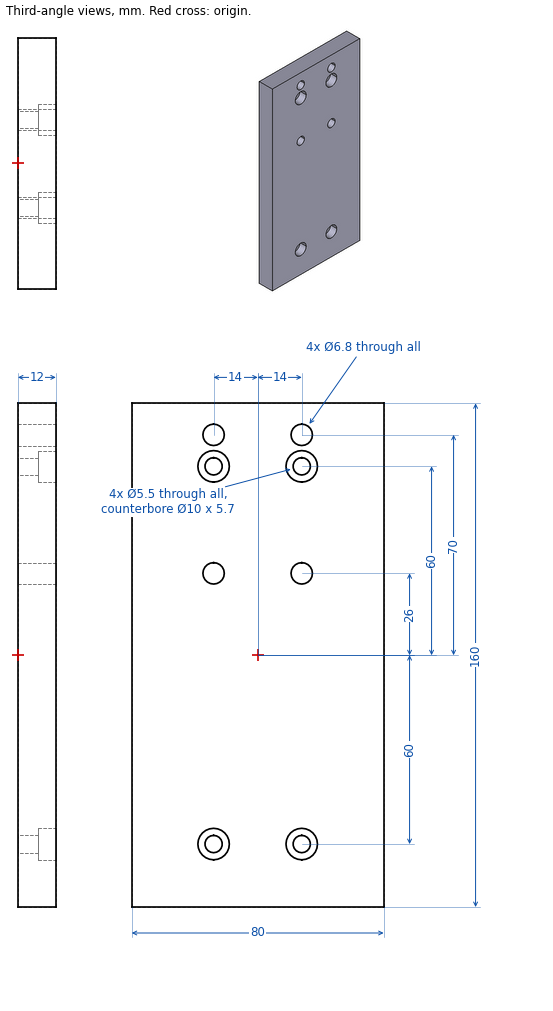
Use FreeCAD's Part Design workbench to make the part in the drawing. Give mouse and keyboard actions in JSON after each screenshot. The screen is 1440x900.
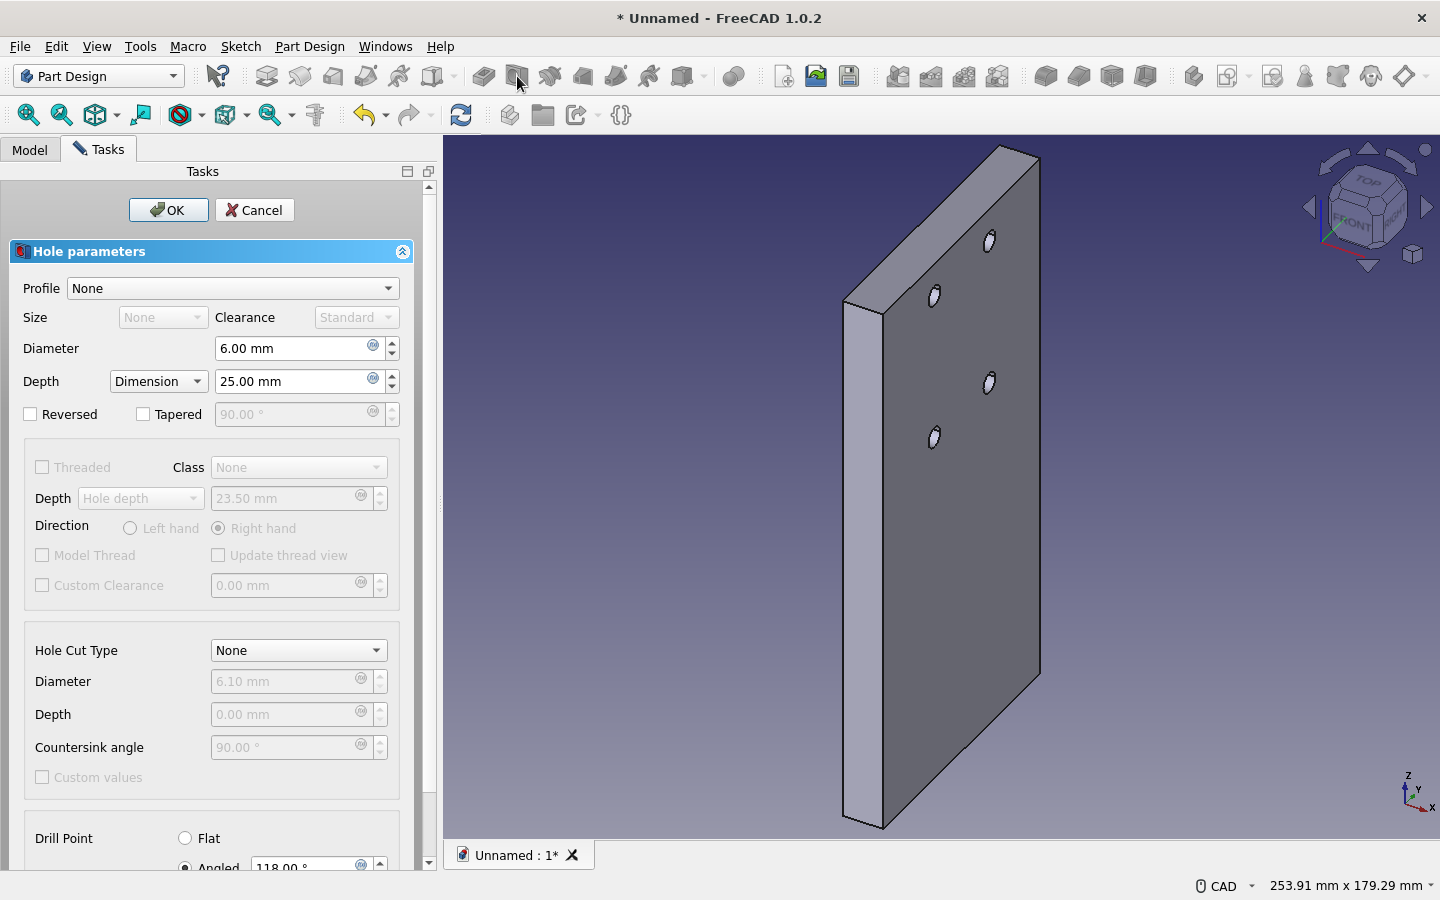
{"action": "triple_click", "coordinate": [300, 348]}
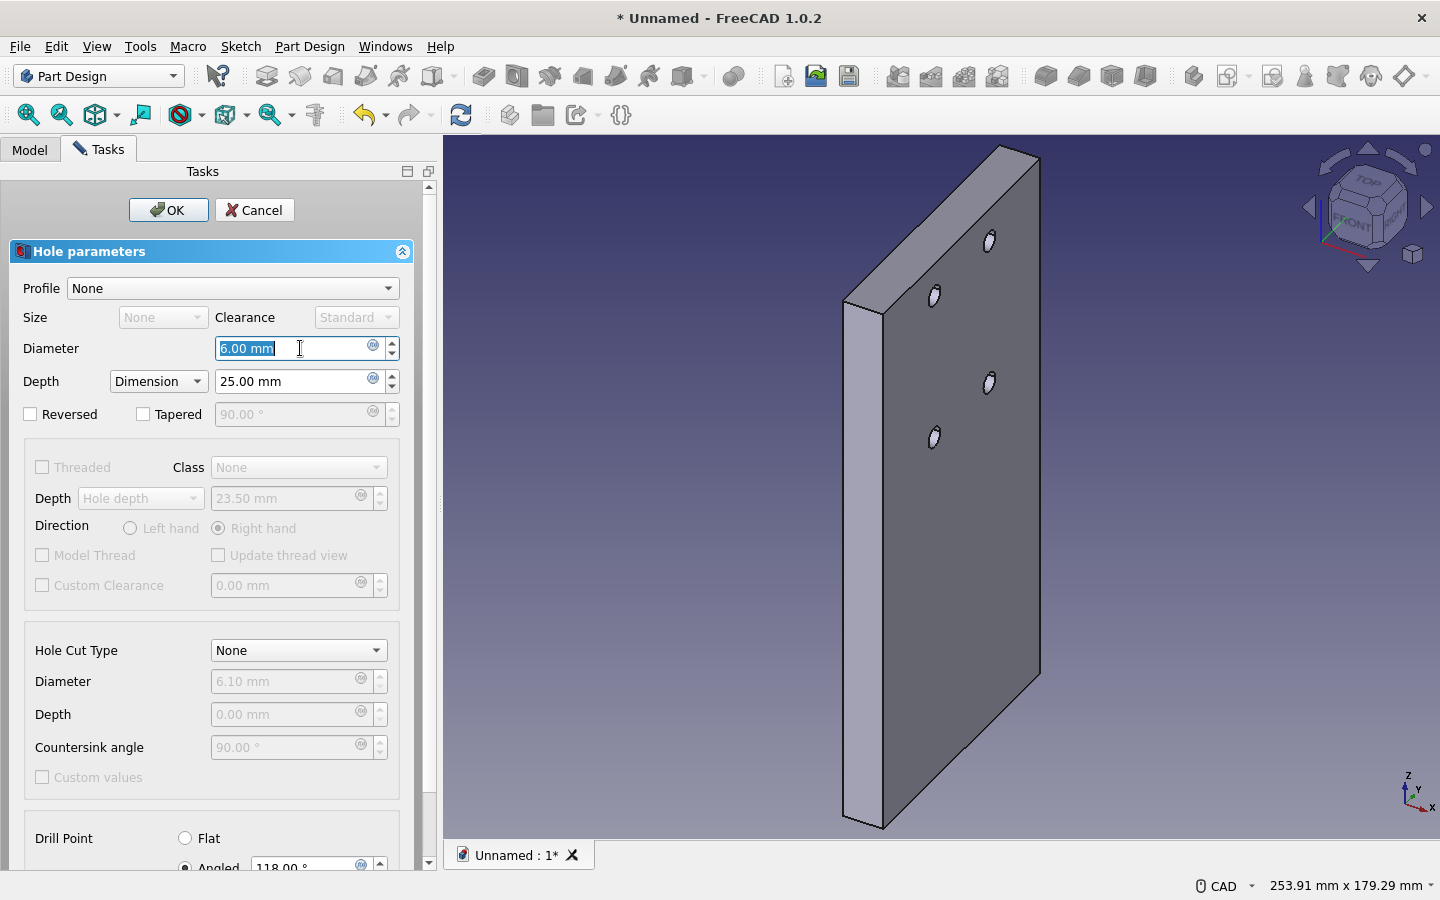
{"action": "type", "text": "6.8"}
{"action": "key", "text": "Tab"}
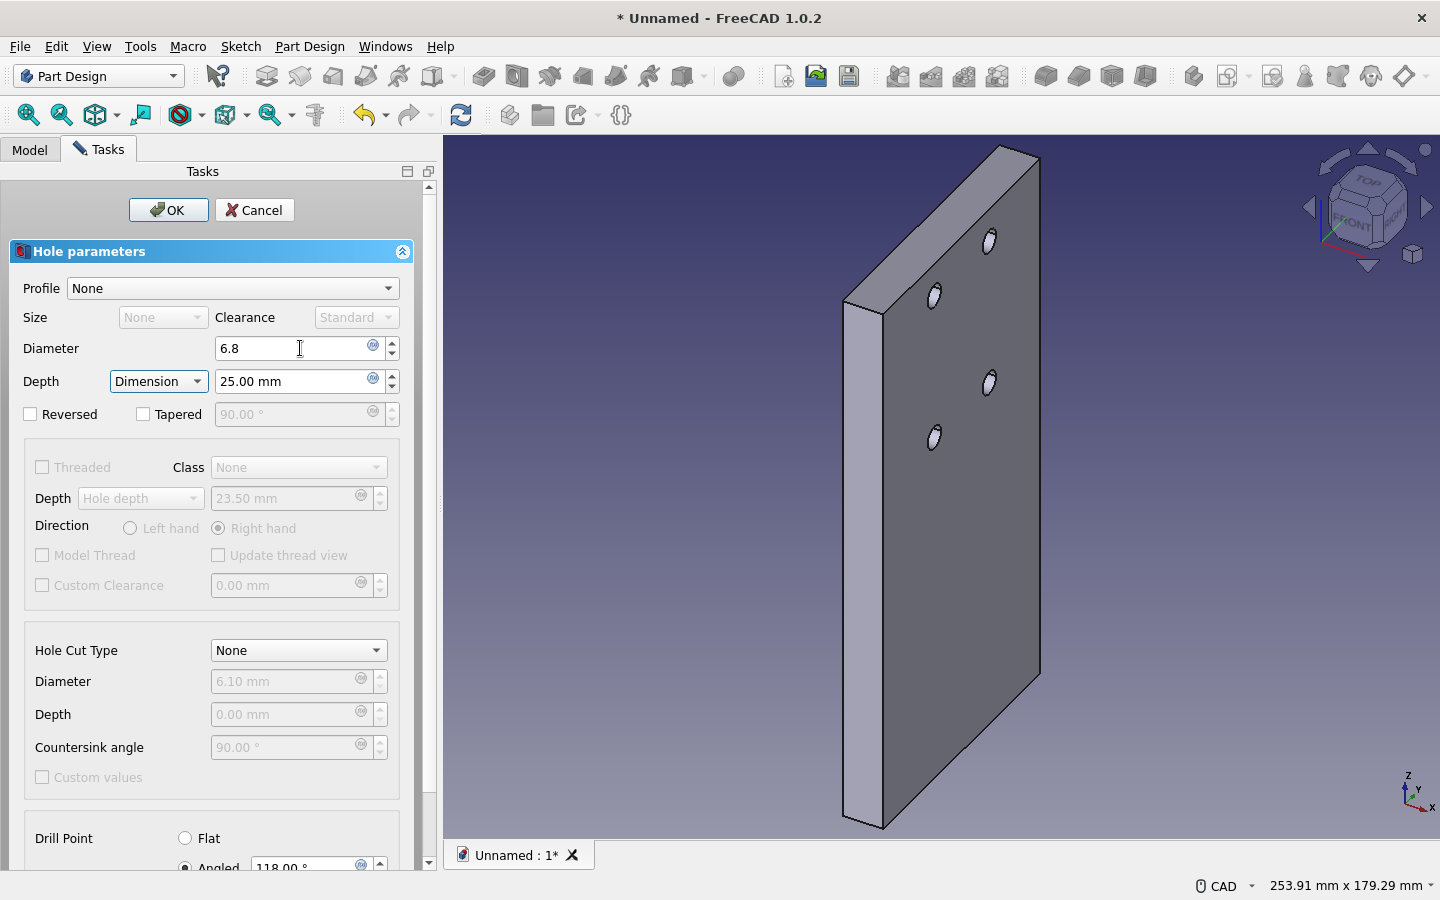
{"action": "left_click", "coordinate": [160, 382]}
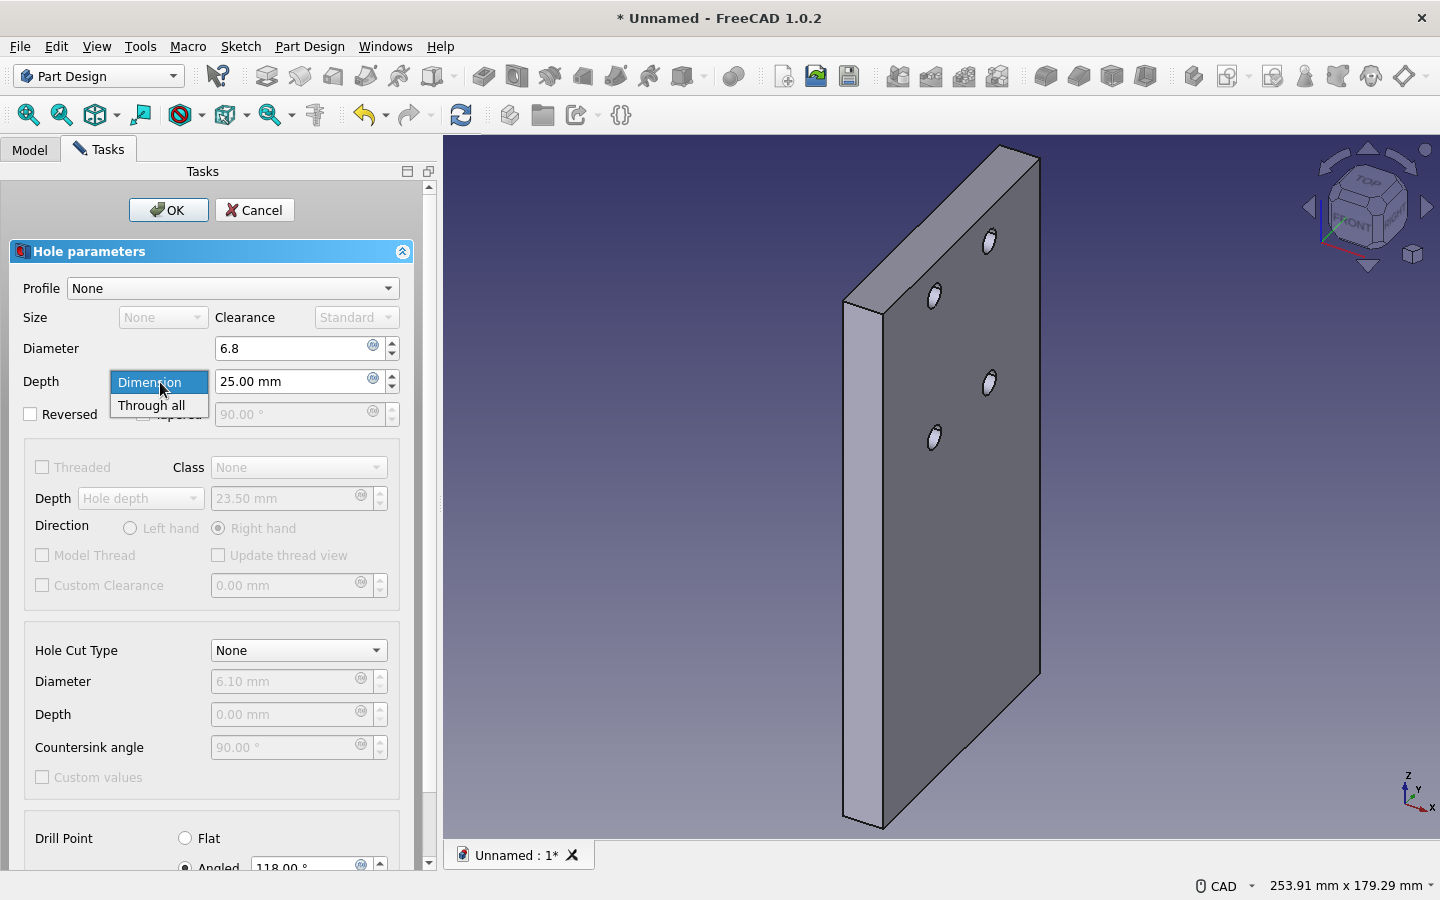
{"action": "left_click", "coordinate": [158, 406]}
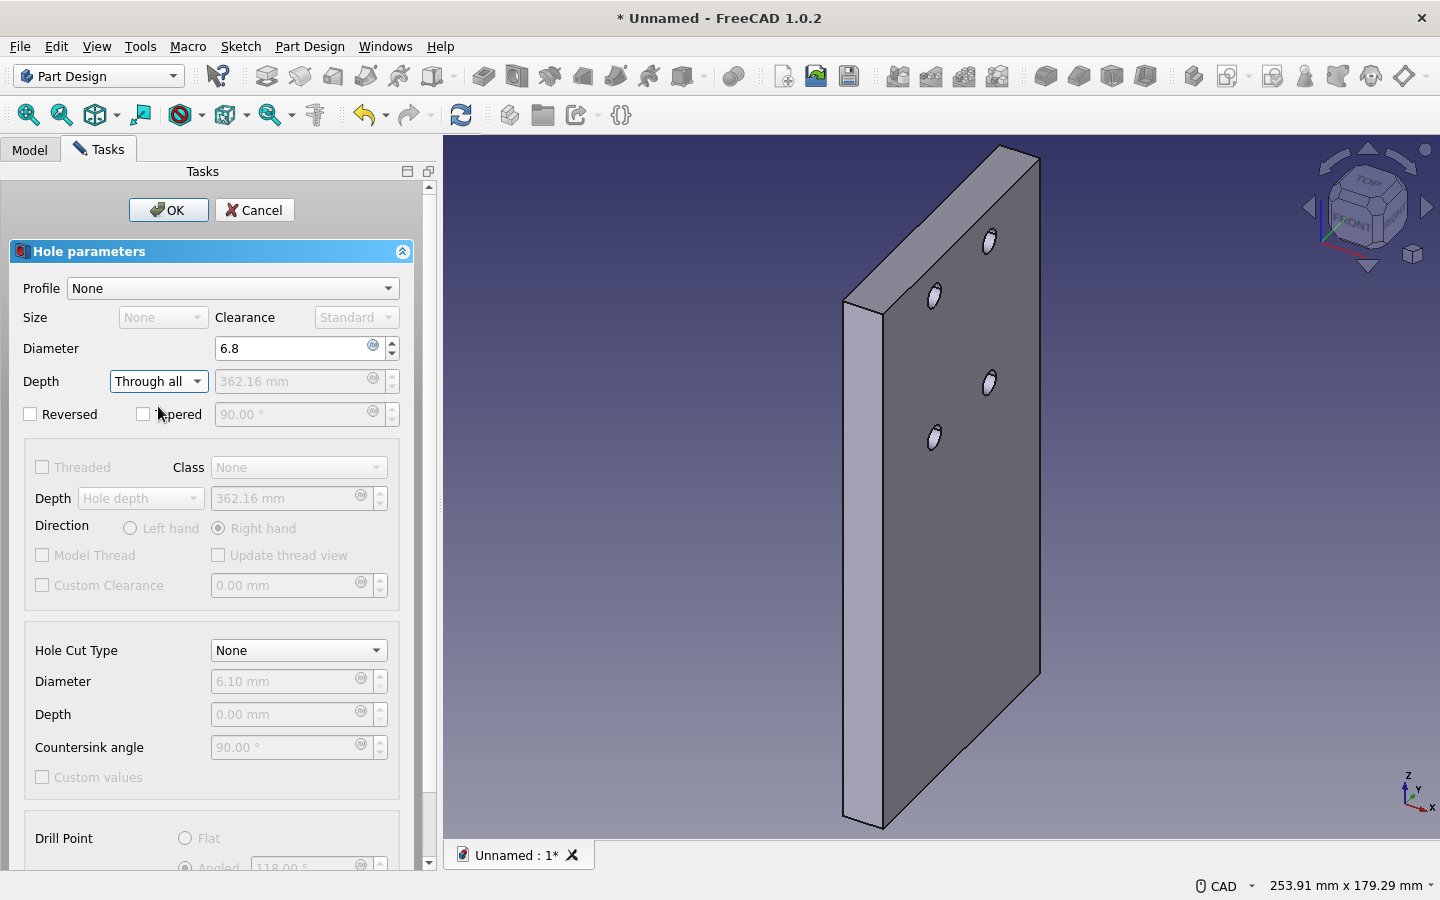
{"action": "left_click", "coordinate": [169, 210]}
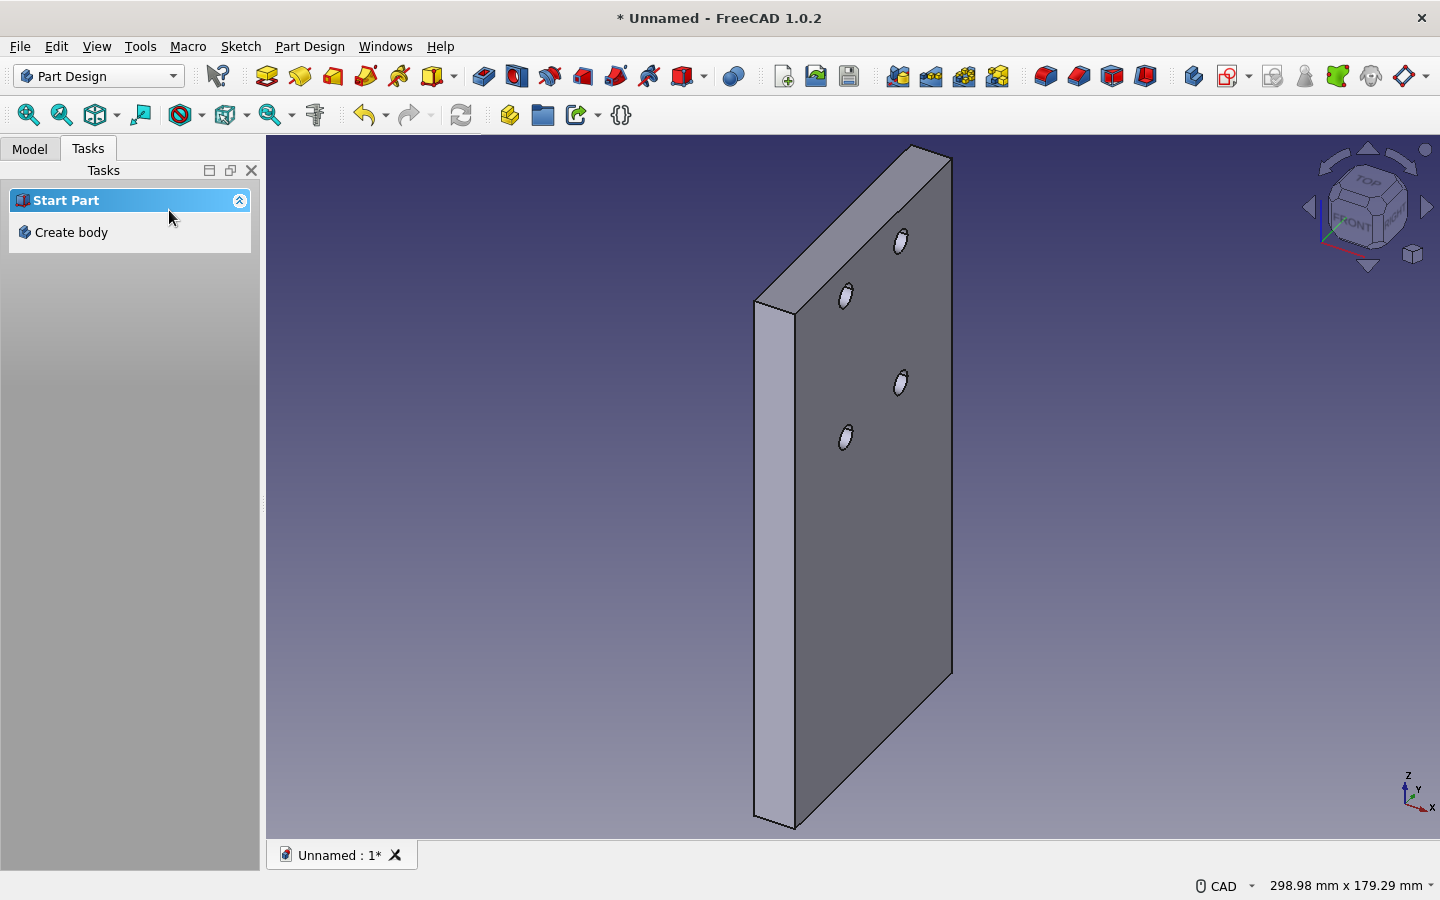
{"action": "left_click", "coordinate": [873, 566]}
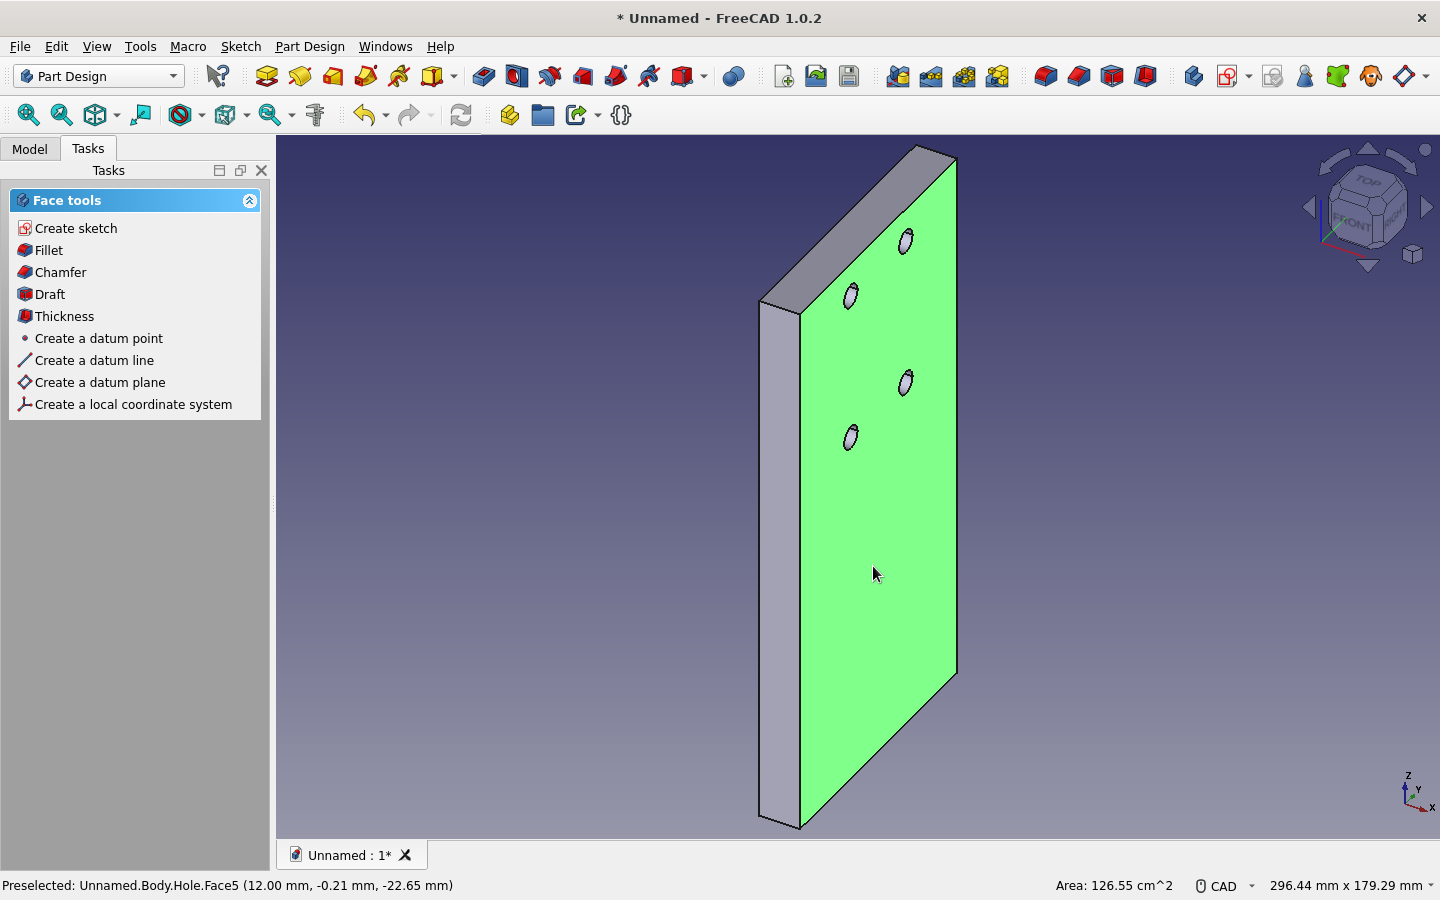
{"action": "left_click", "coordinate": [1226, 76]}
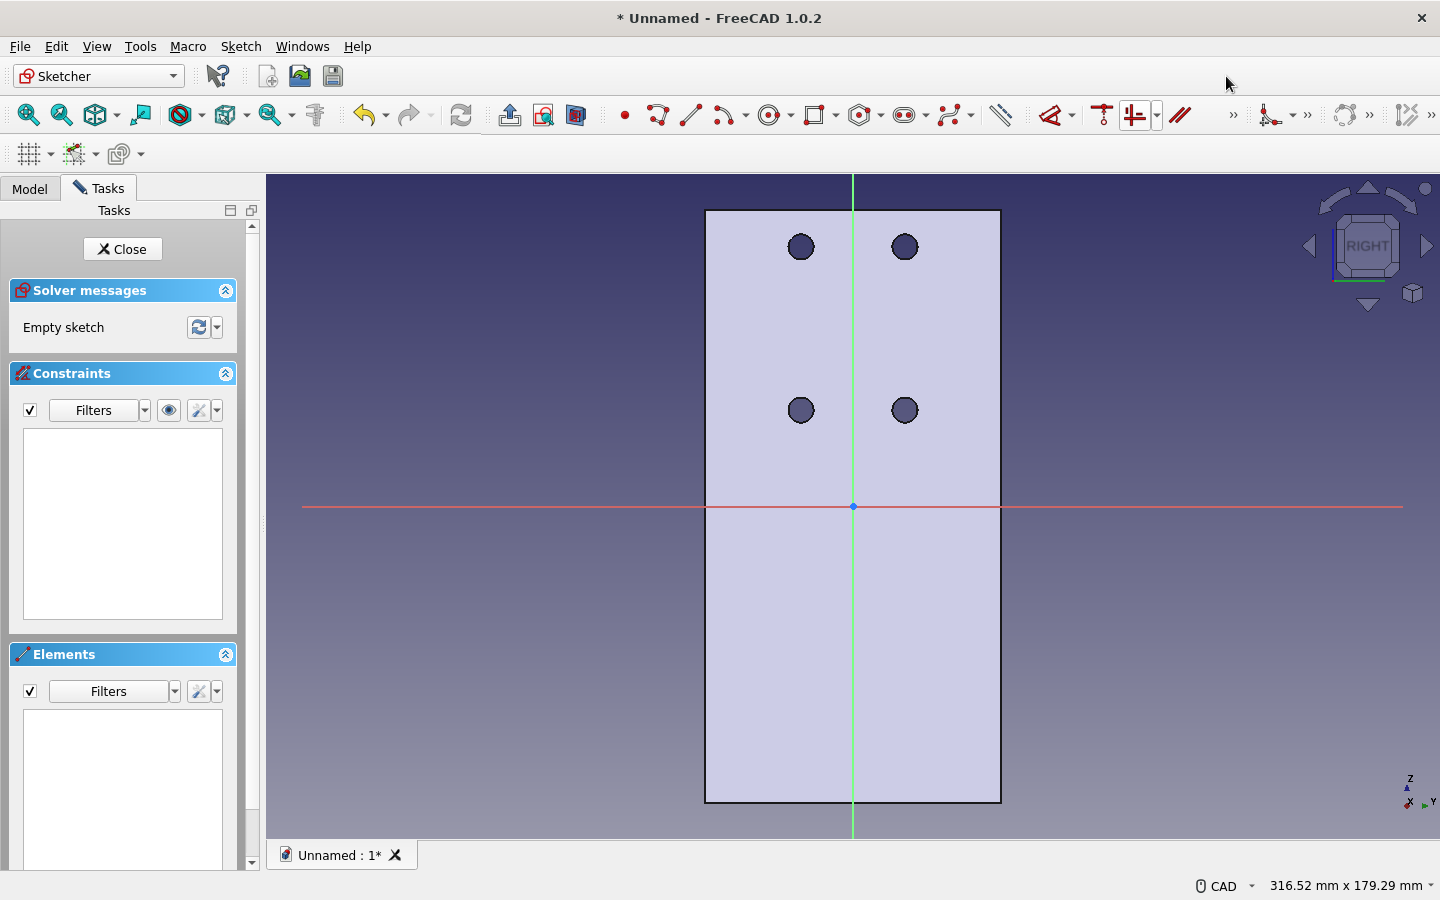
{"action": "left_click", "coordinate": [768, 116]}